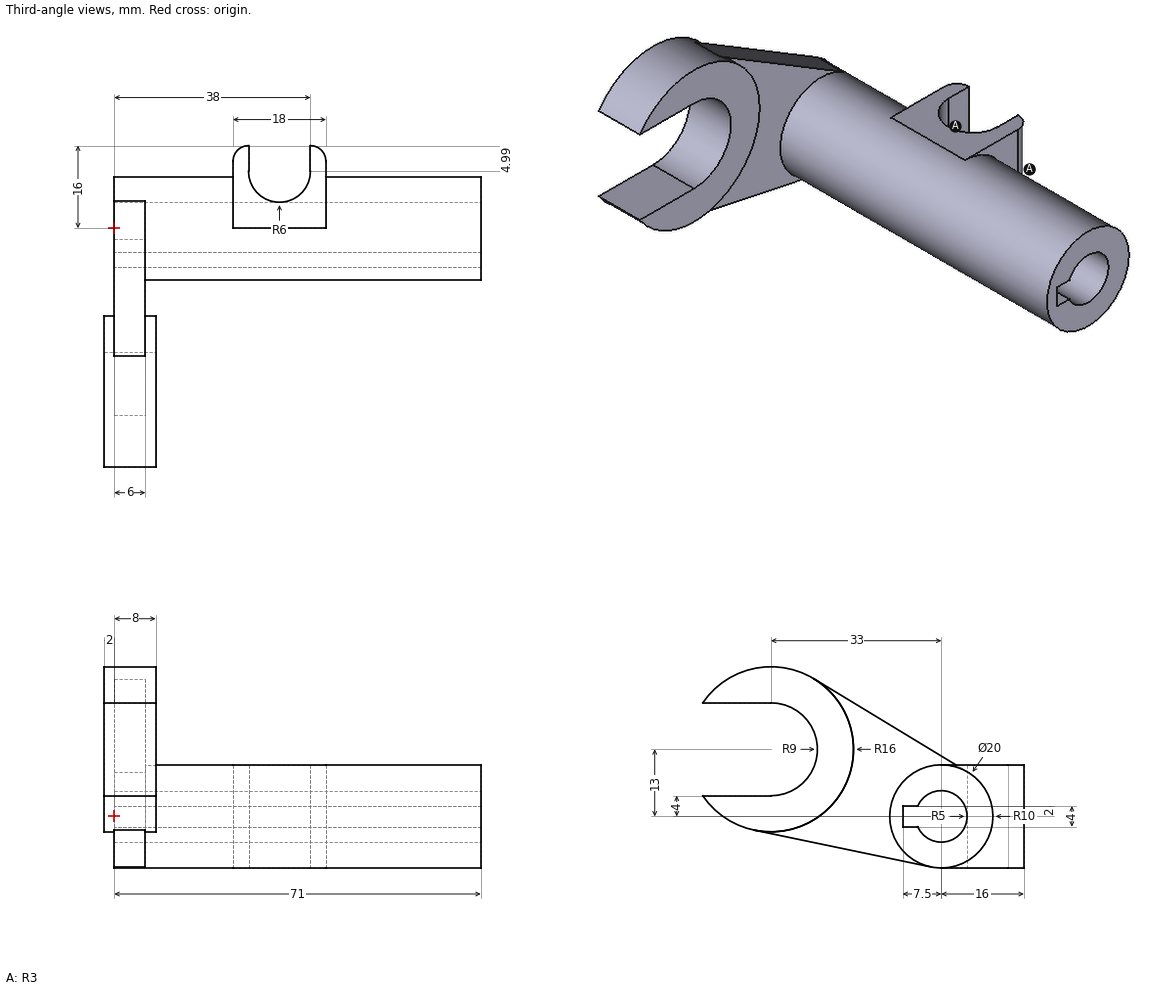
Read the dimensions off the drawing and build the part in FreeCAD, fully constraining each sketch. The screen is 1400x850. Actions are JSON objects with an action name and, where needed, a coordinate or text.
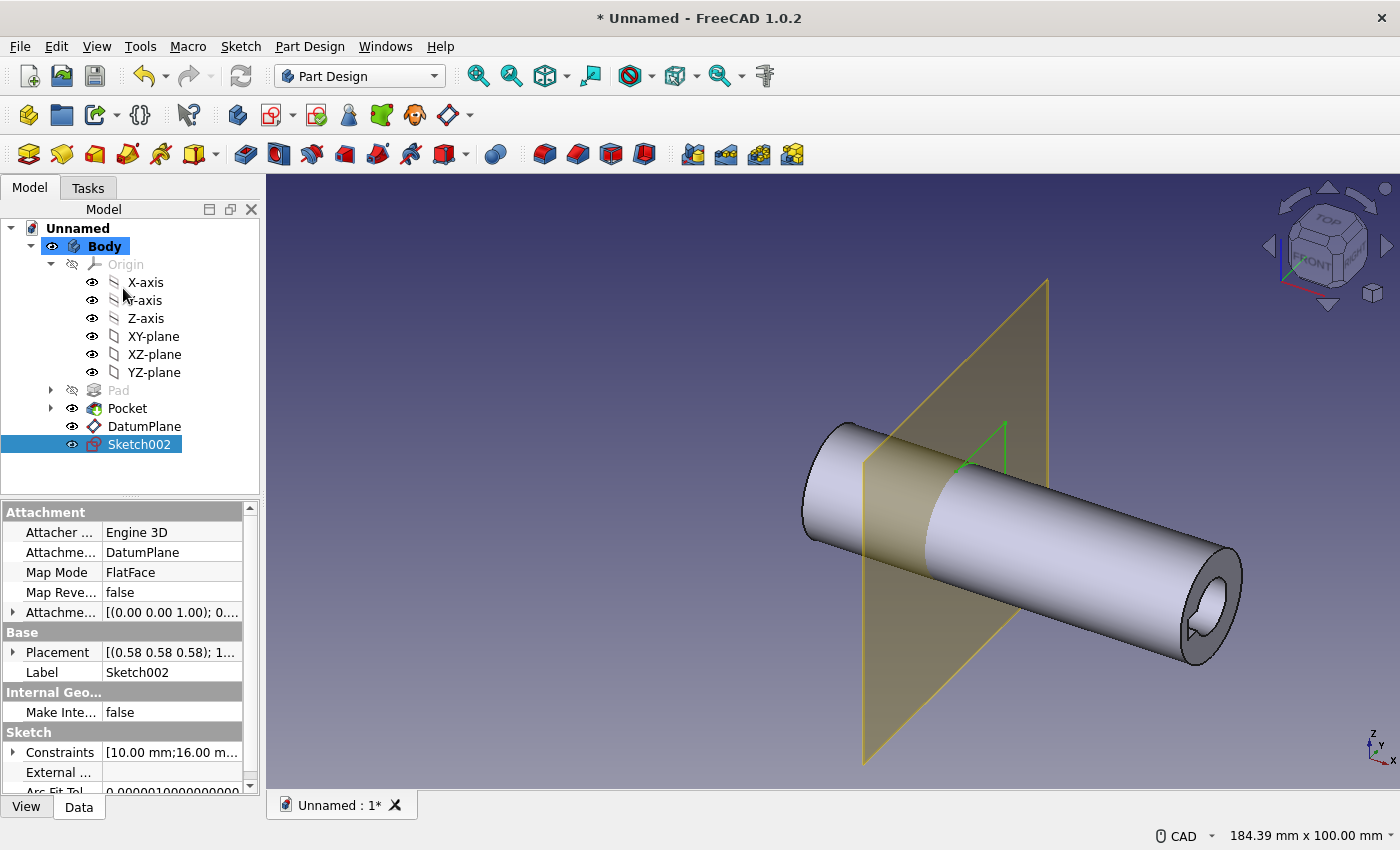
{"action": "left_click", "coordinate": [29, 154]}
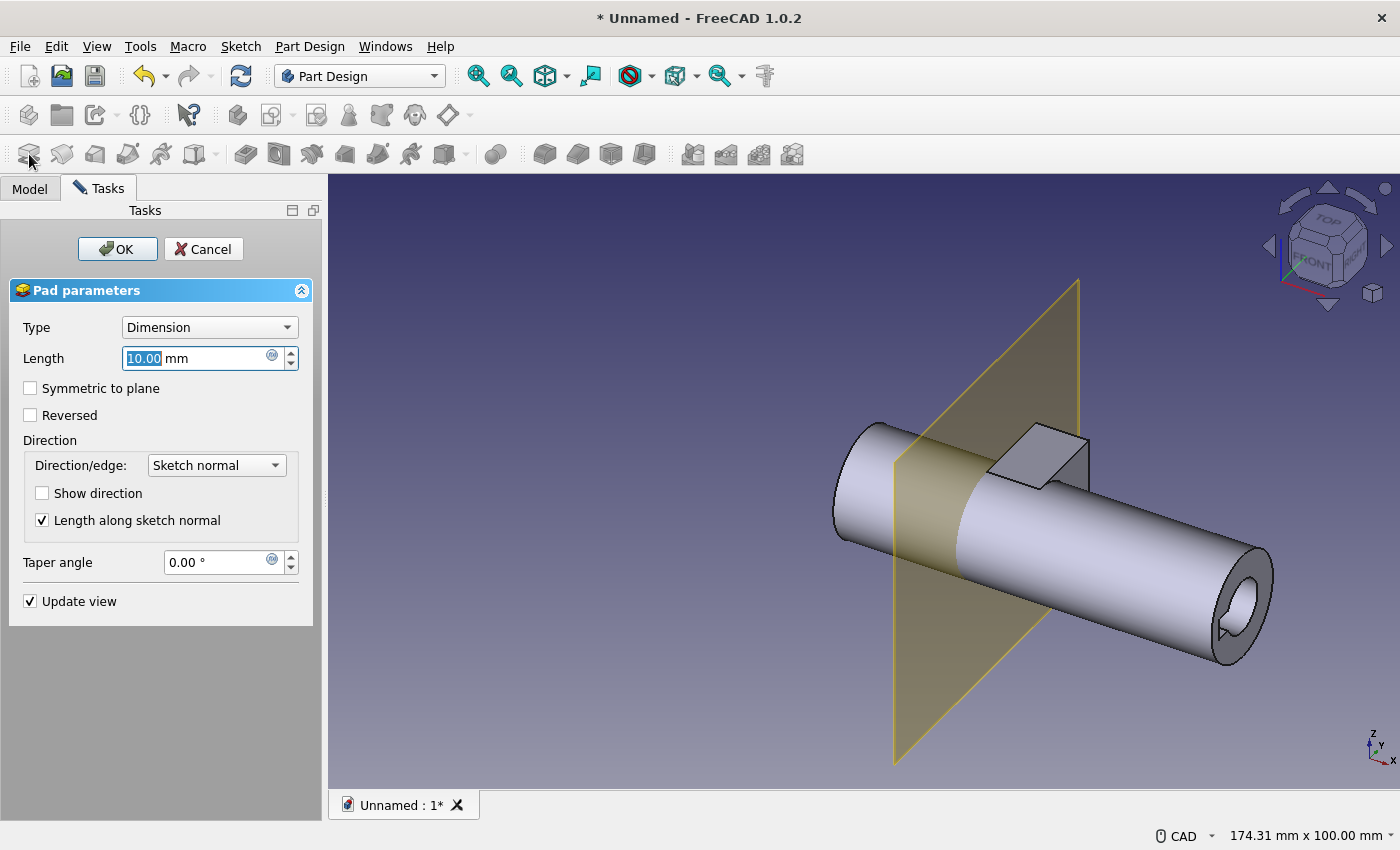
{"action": "type", "text": "18"}
{"action": "key", "text": "Tab"}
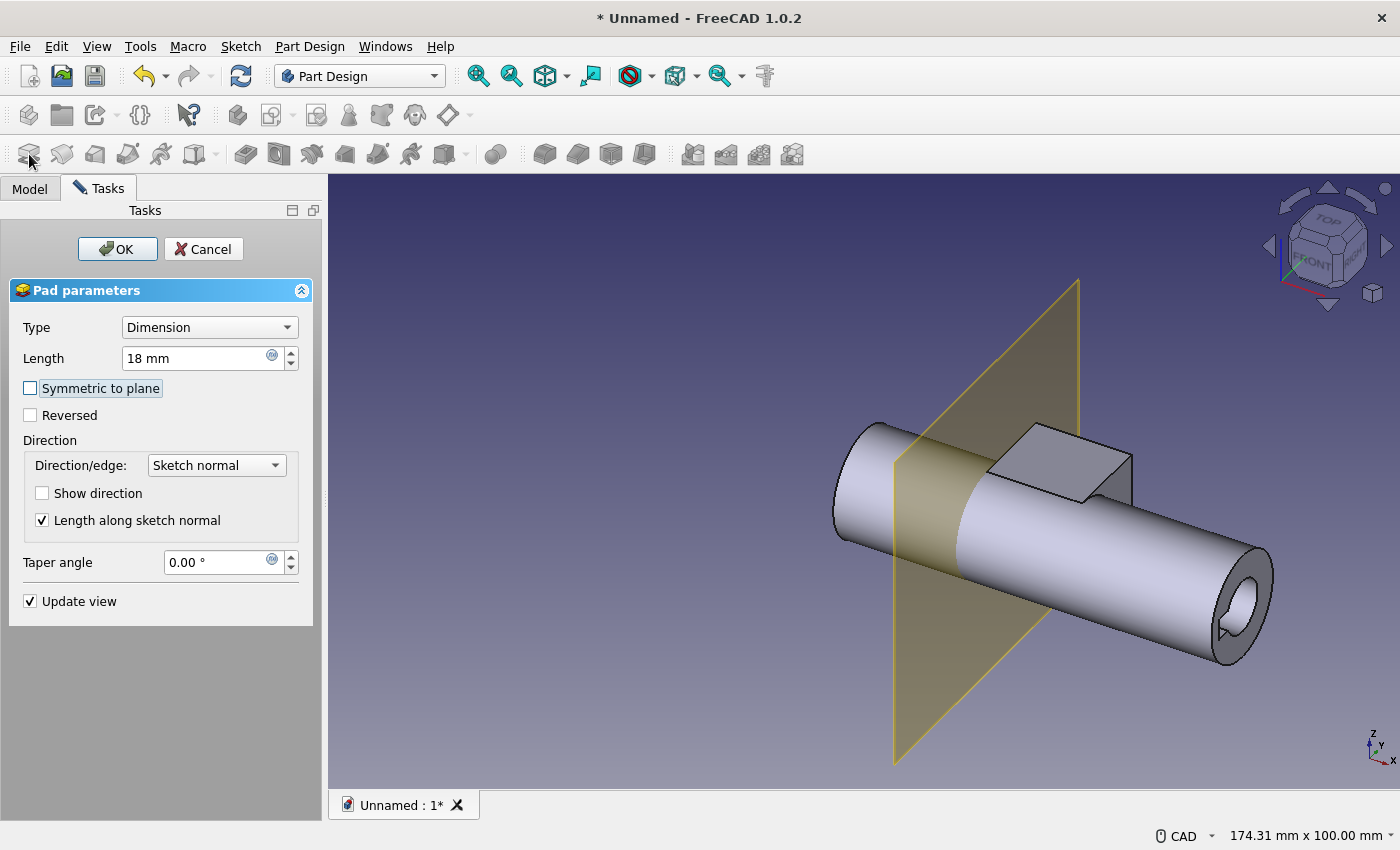
{"action": "left_click", "coordinate": [118, 249]}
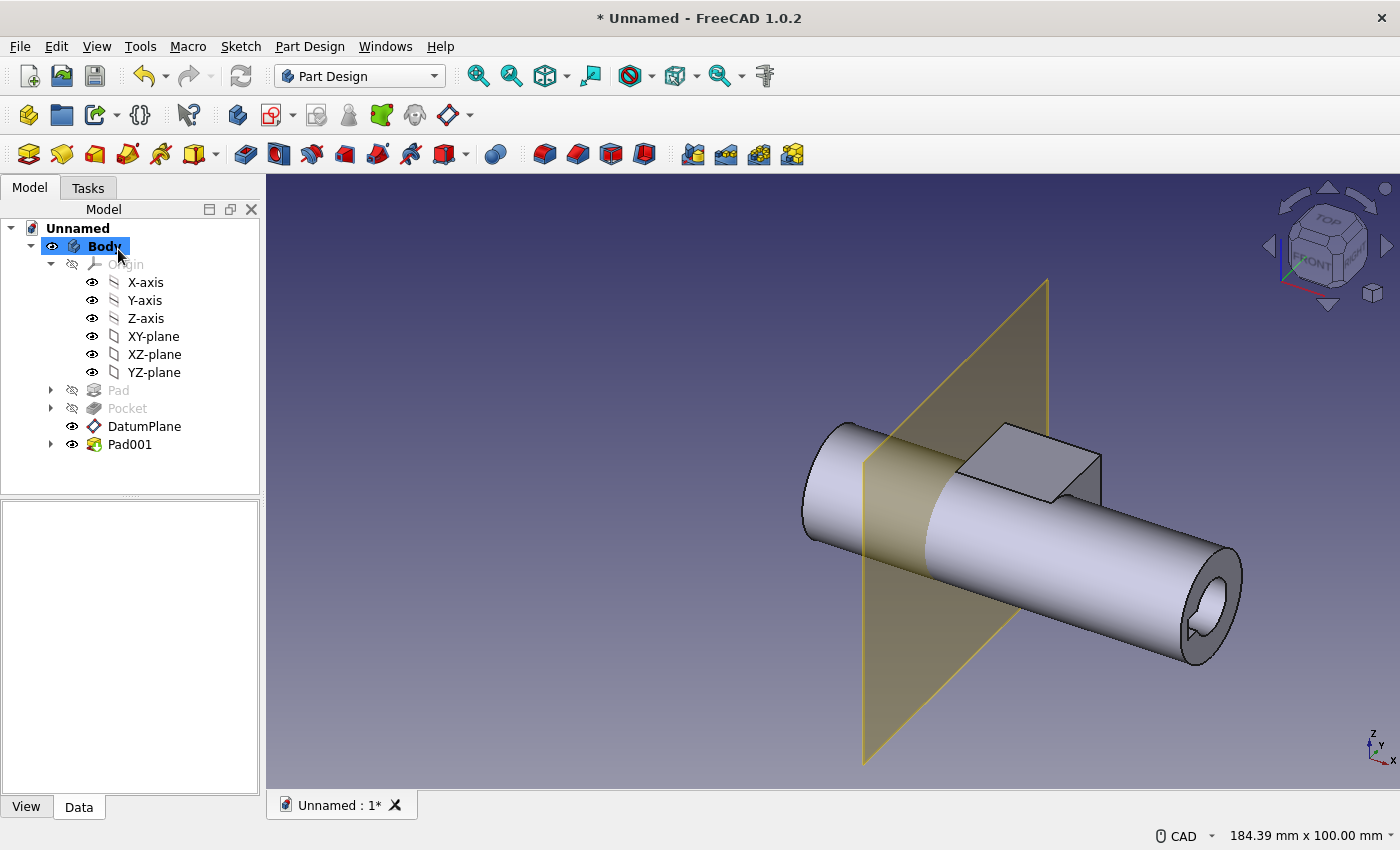
{"action": "left_click", "coordinate": [117, 426]}
{"action": "key", "text": "space"}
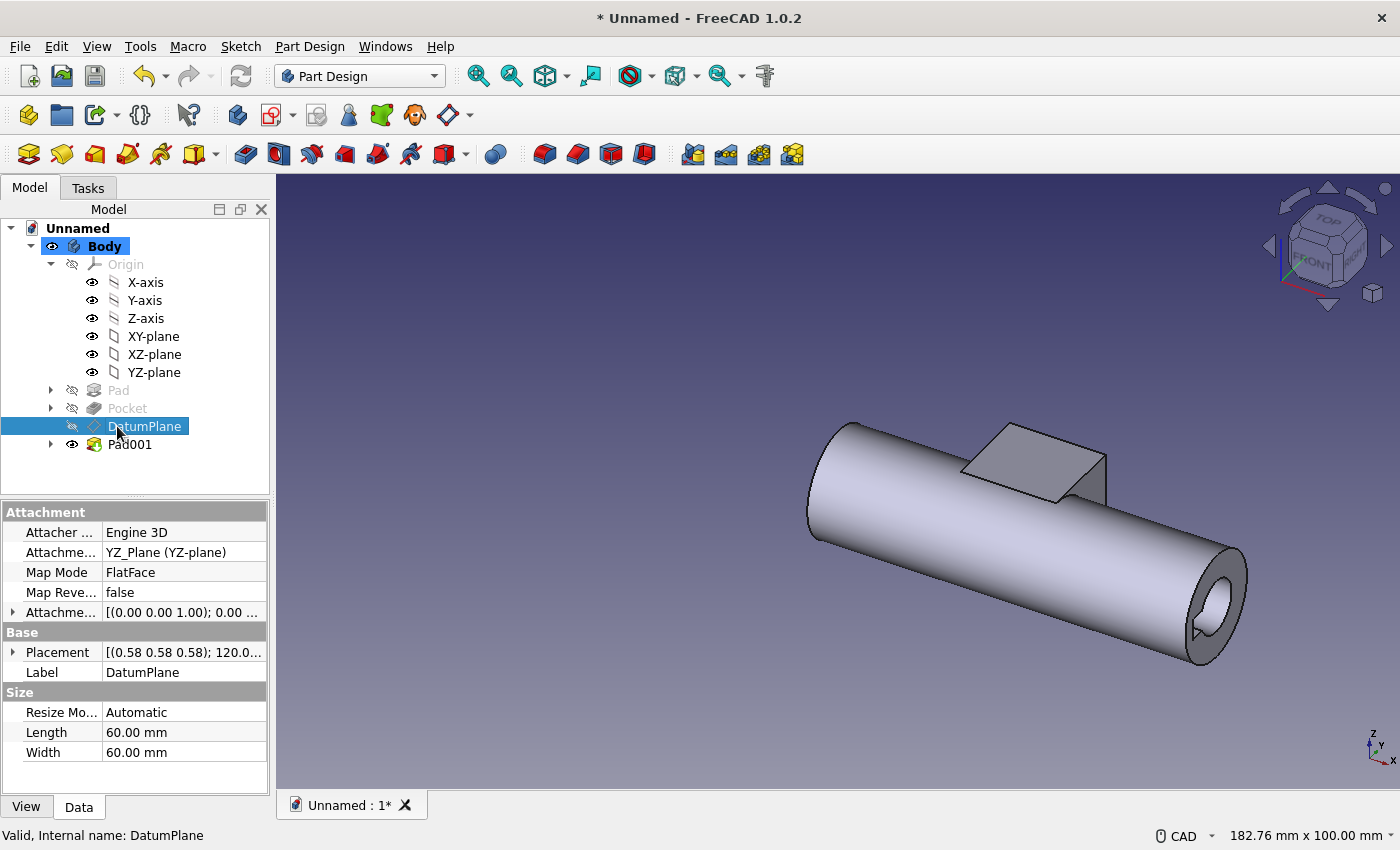
{"action": "key", "text": "0"}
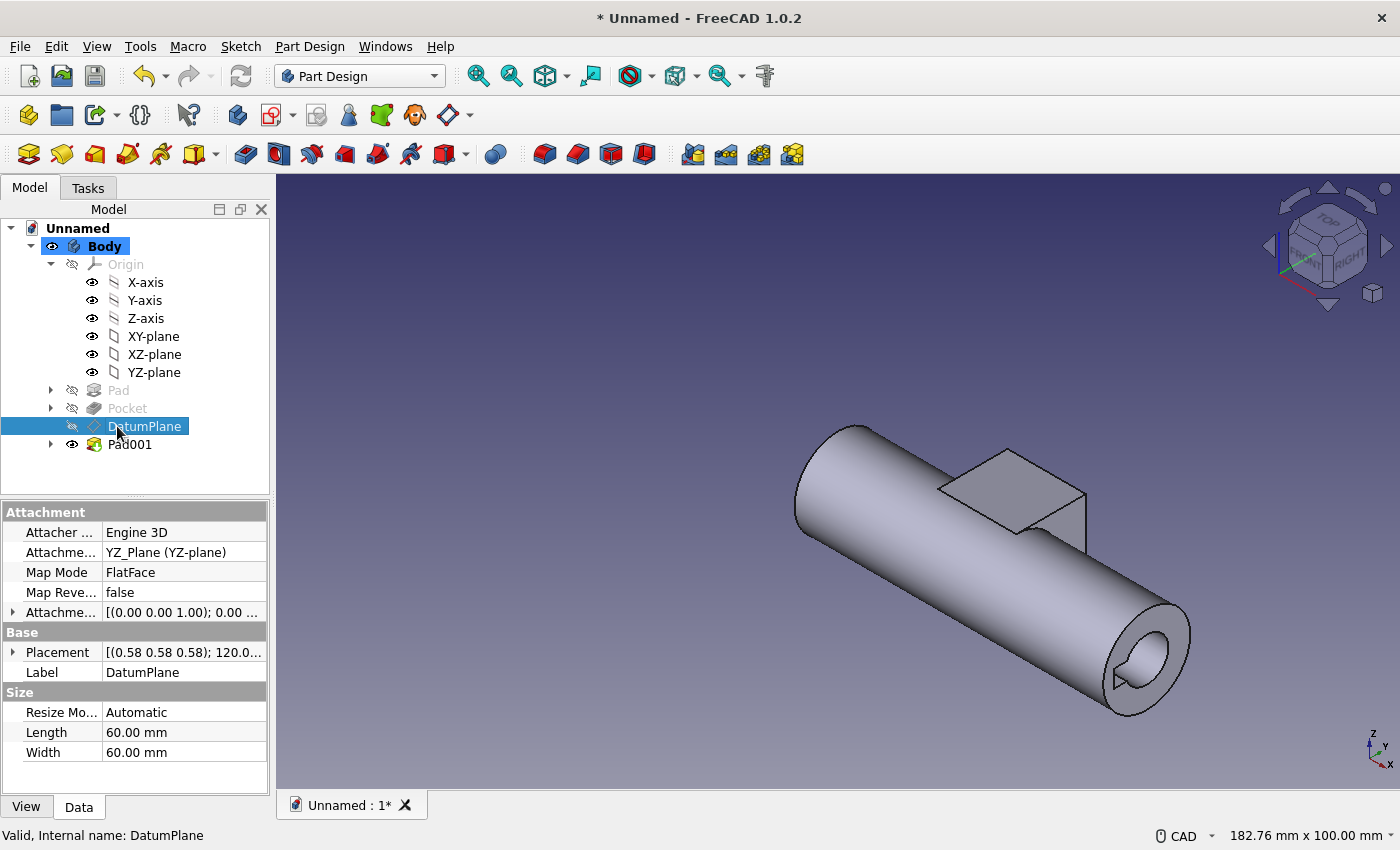
{"action": "key", "text": "2"}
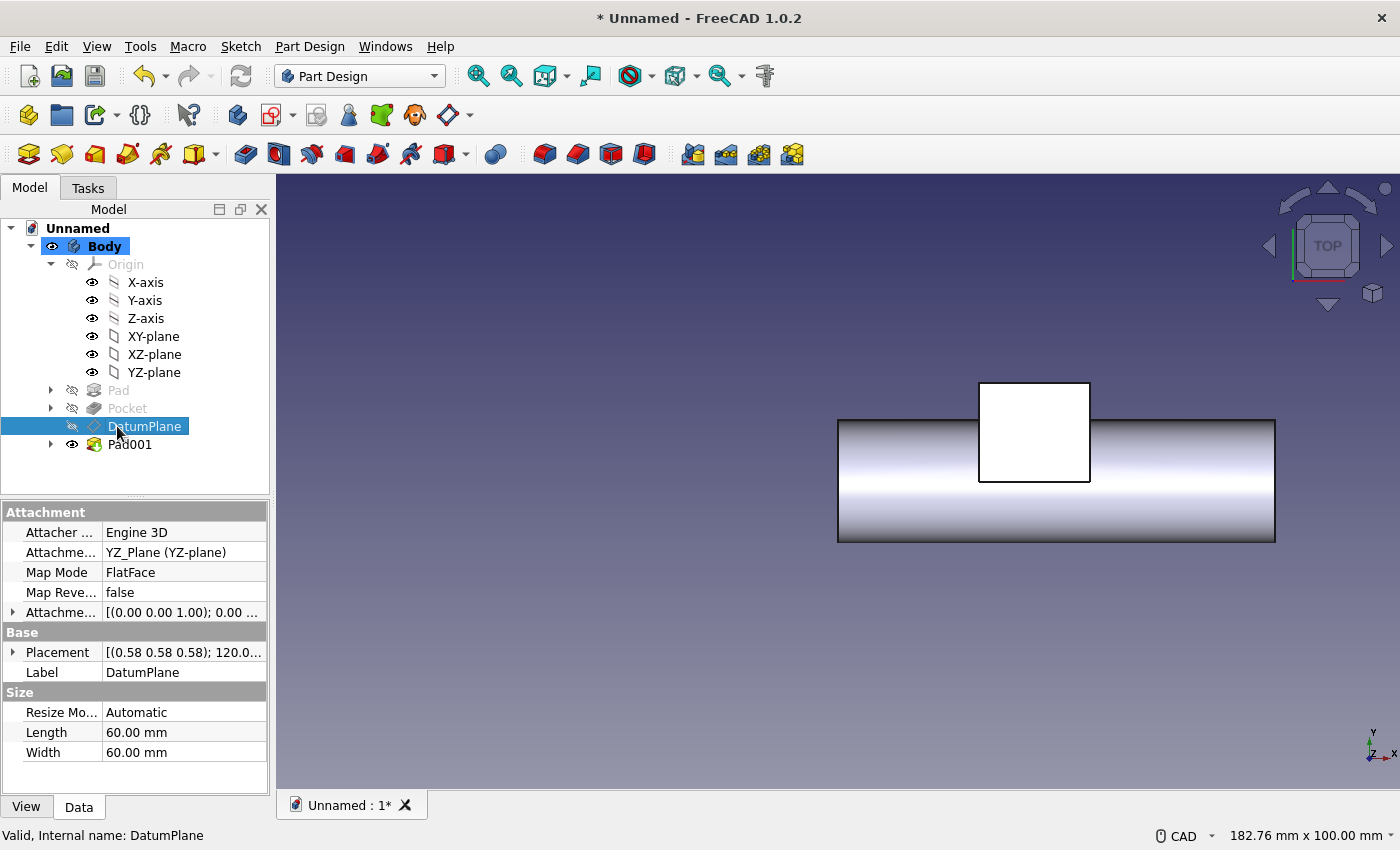
{"action": "key", "text": "v f"}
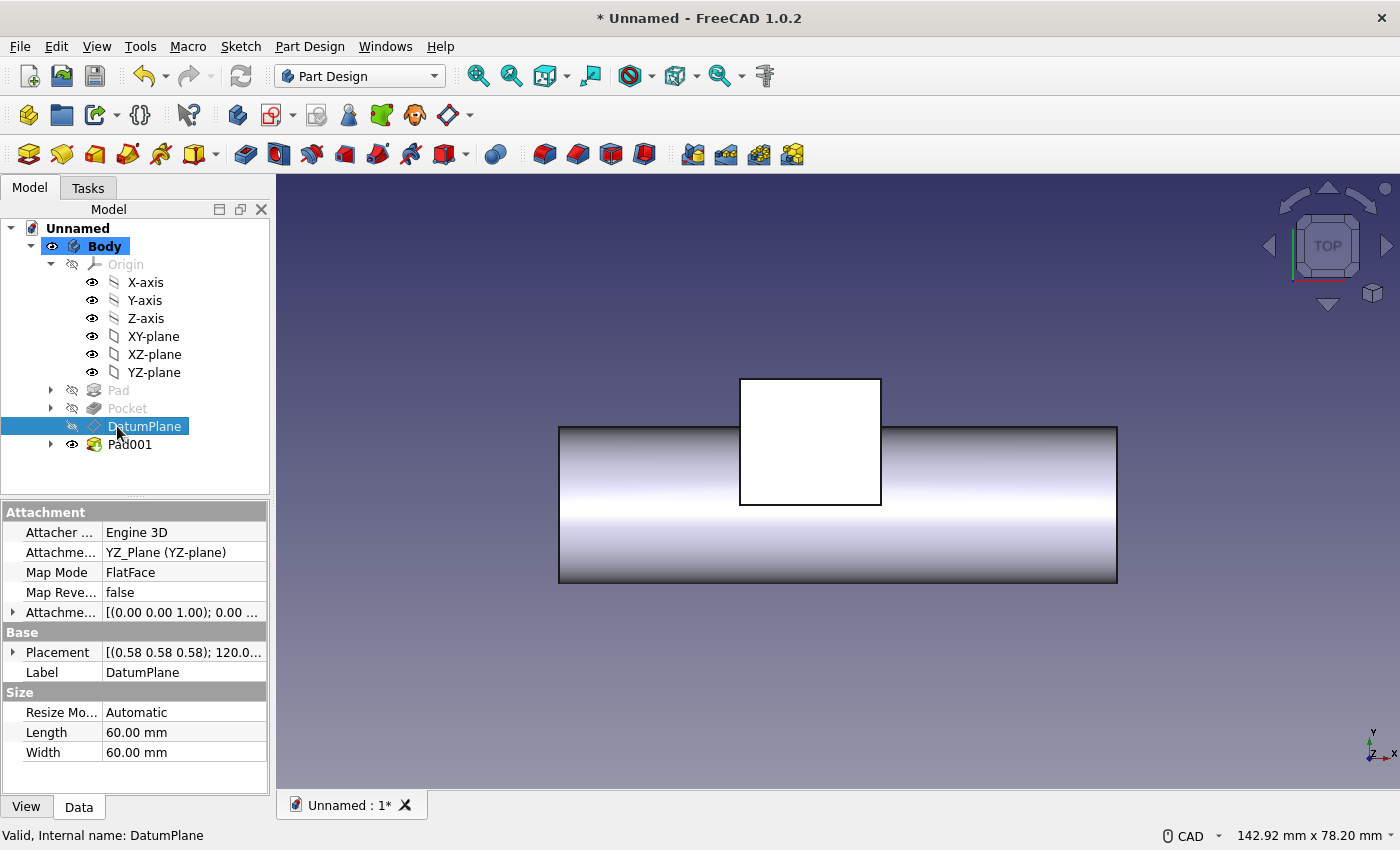
{"action": "key", "text": "1"}